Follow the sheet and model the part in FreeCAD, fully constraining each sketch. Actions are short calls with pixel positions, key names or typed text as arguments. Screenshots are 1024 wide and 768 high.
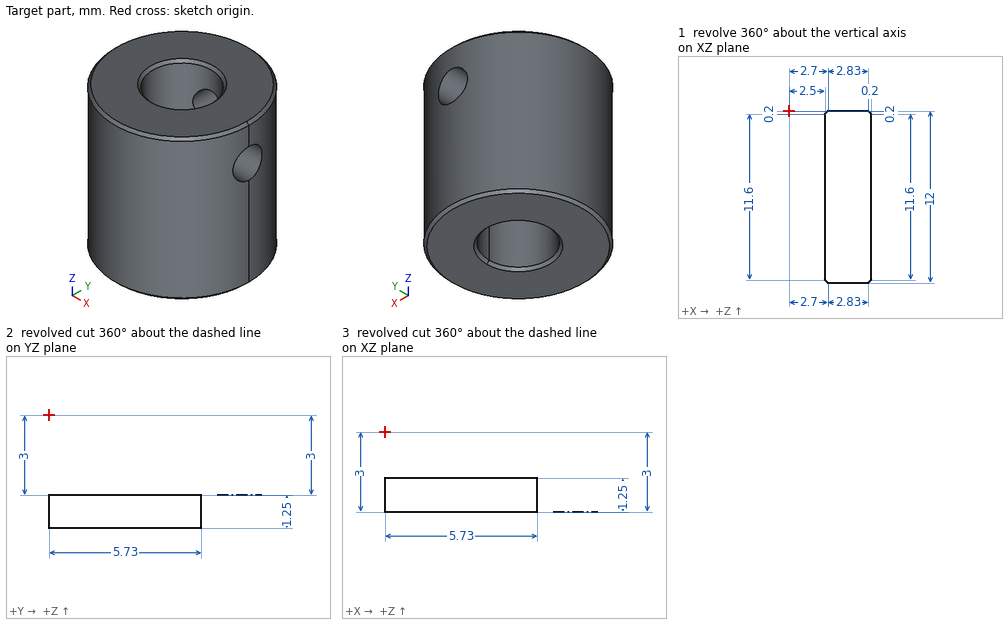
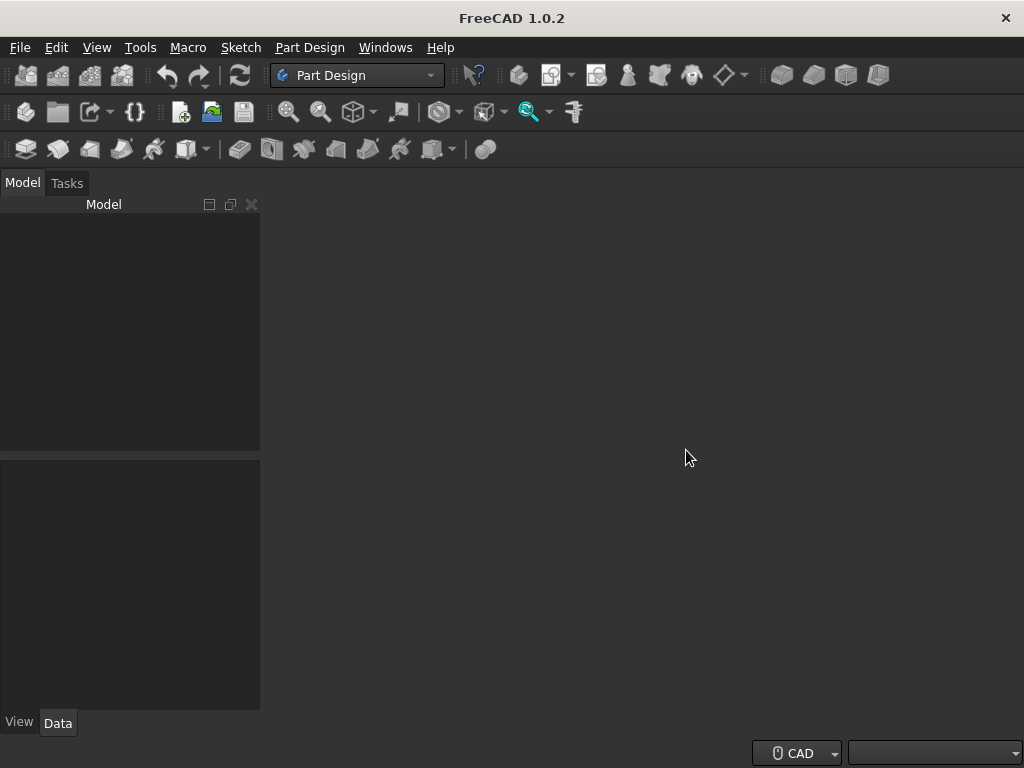
key(ctrl+n)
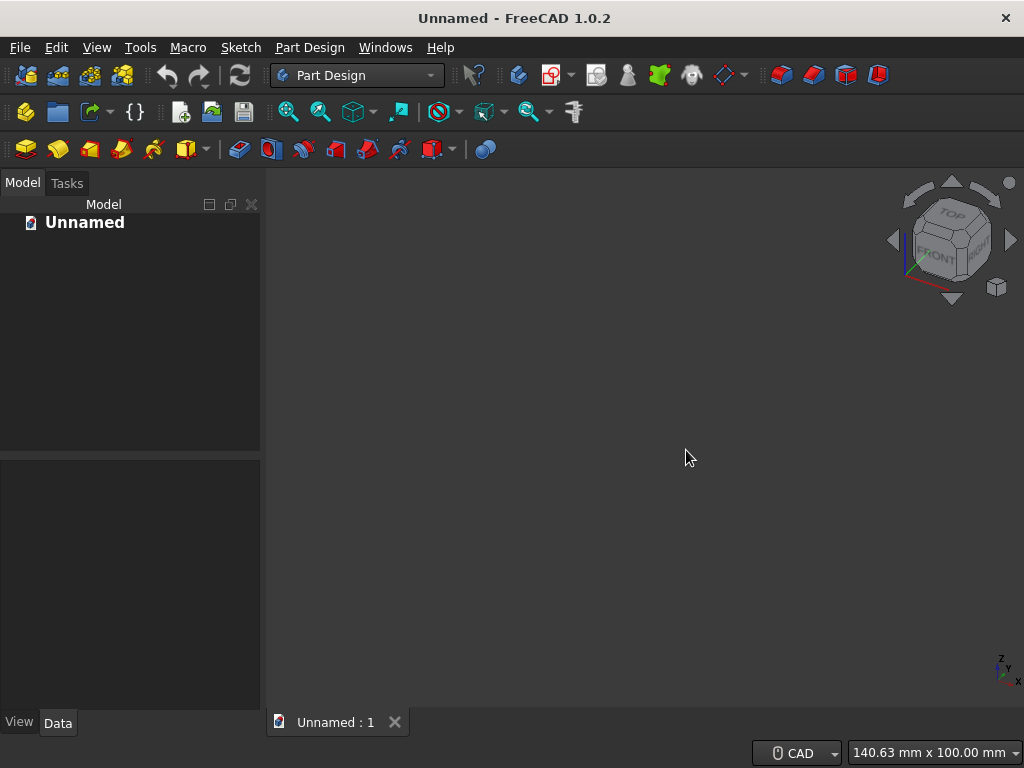
click(552, 76)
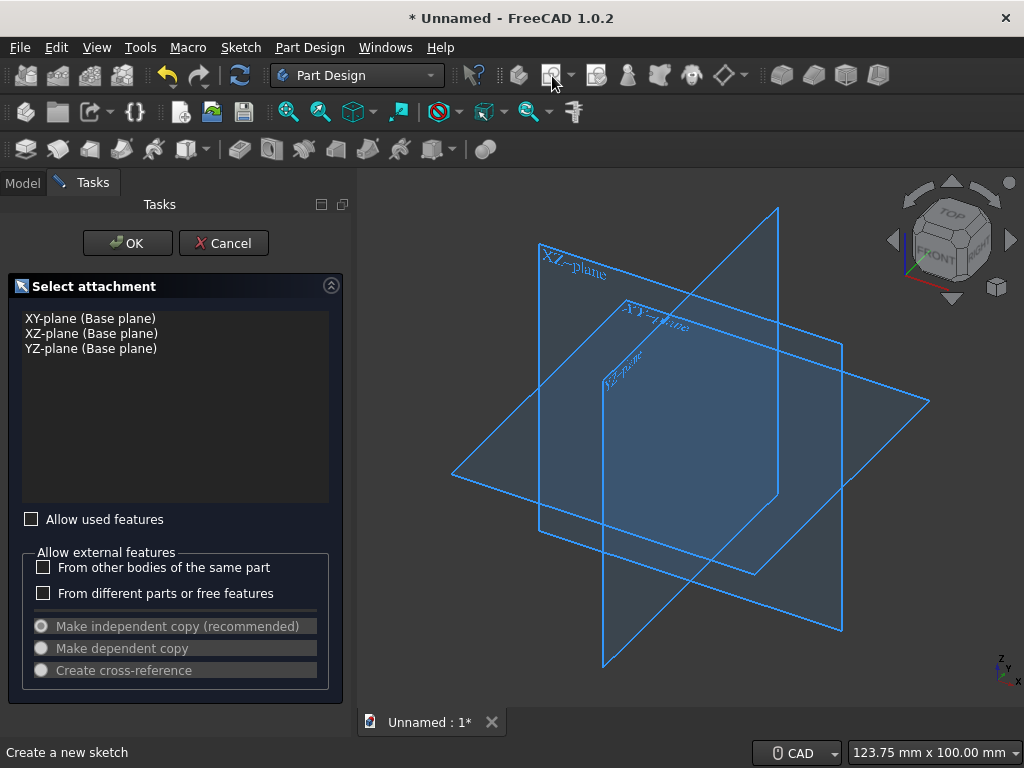
click(82, 334)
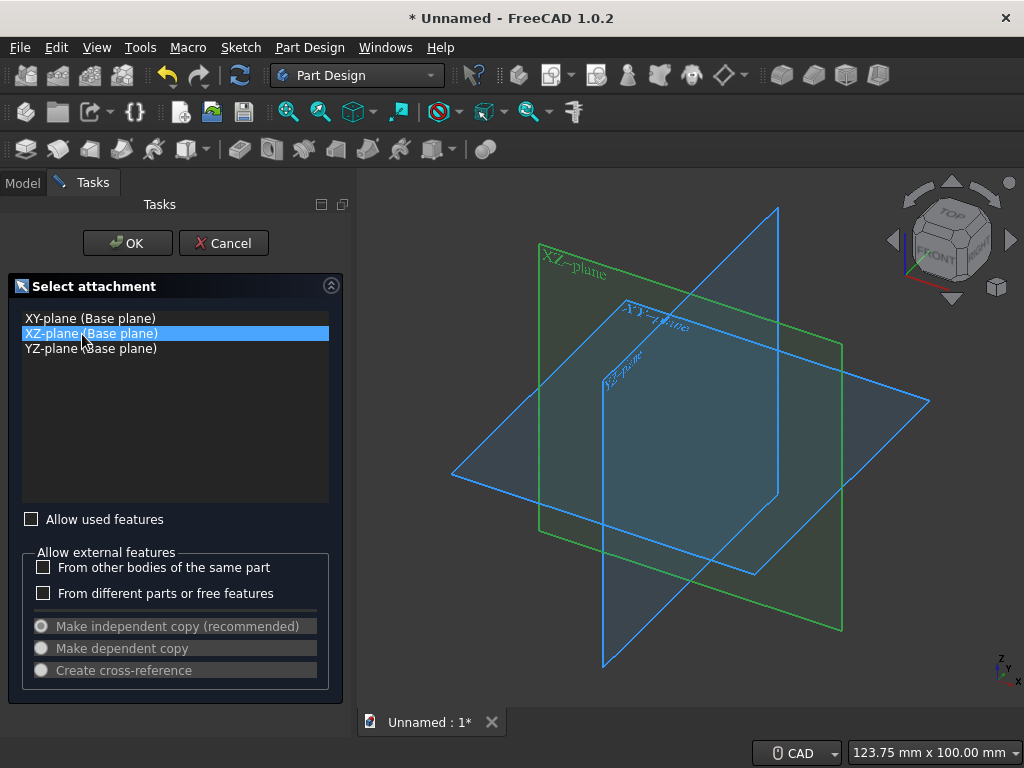
click(128, 243)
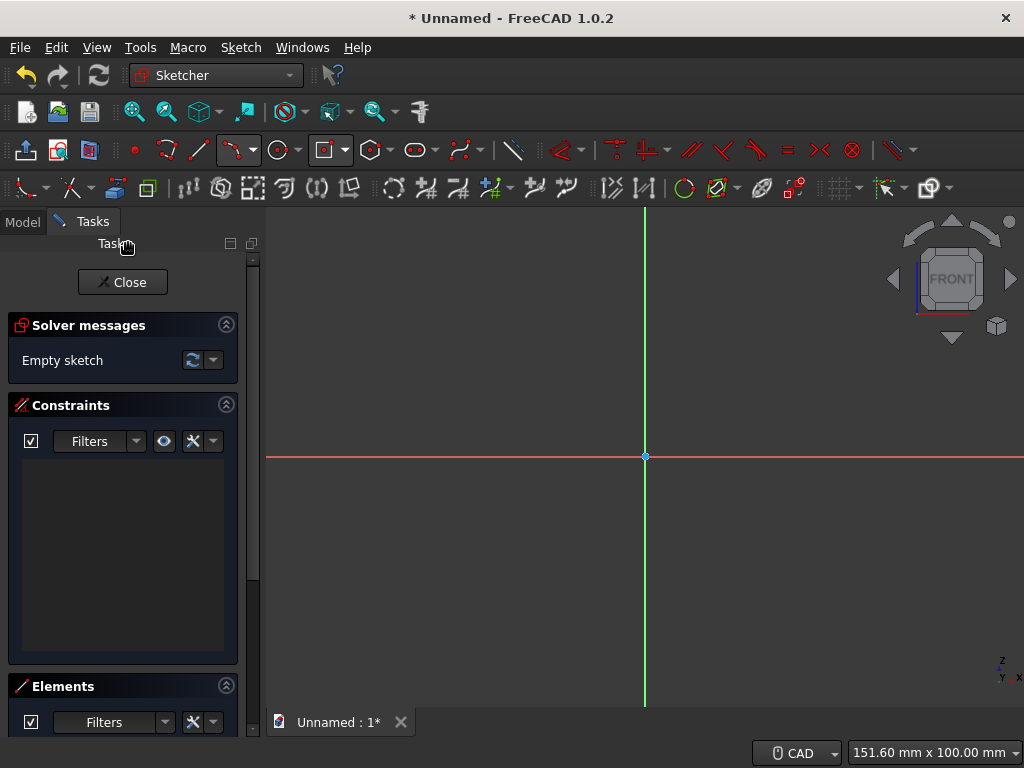
scroll(680, 495, up, 8)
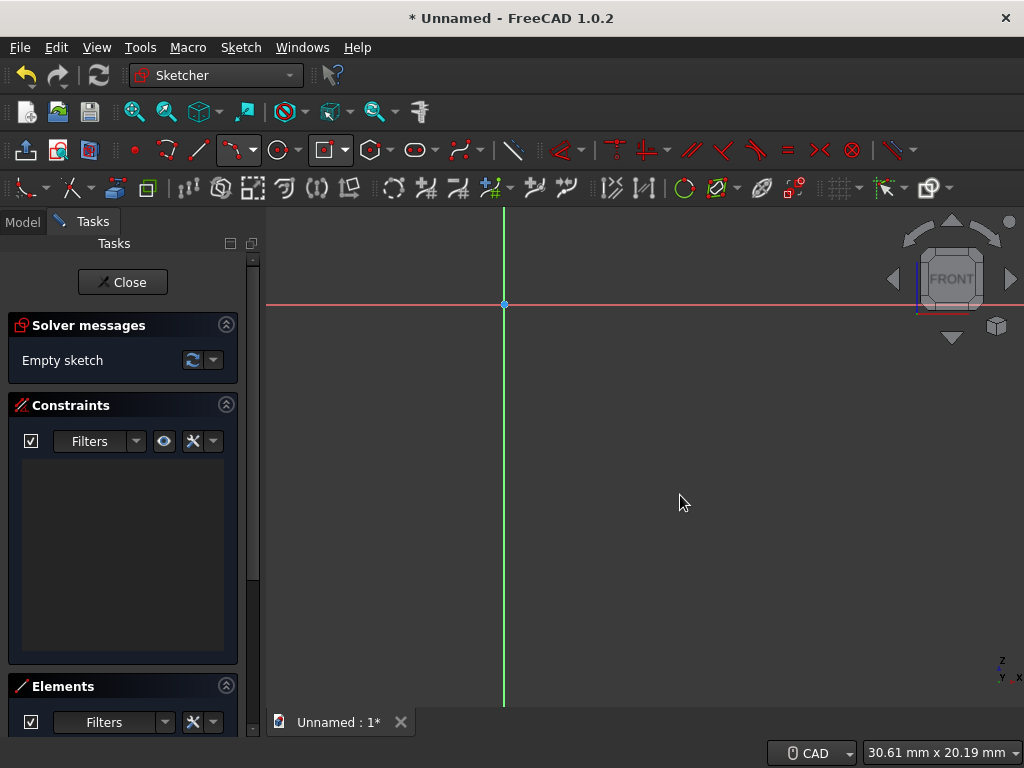
click(168, 150)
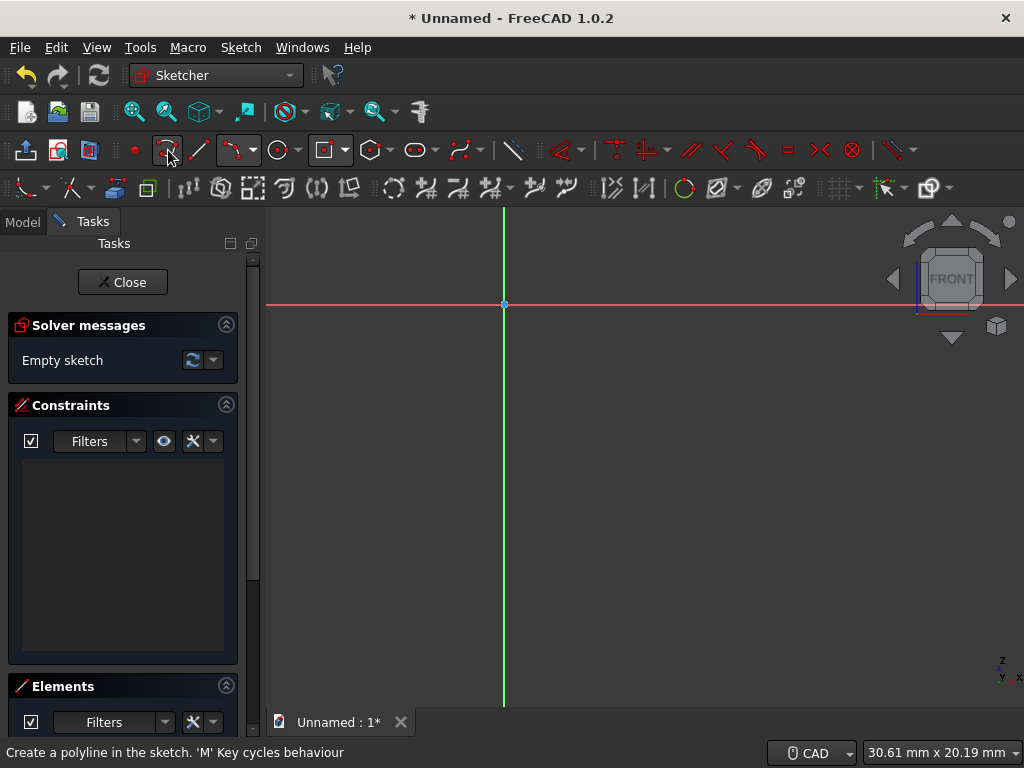
scroll(566, 309, up, 6)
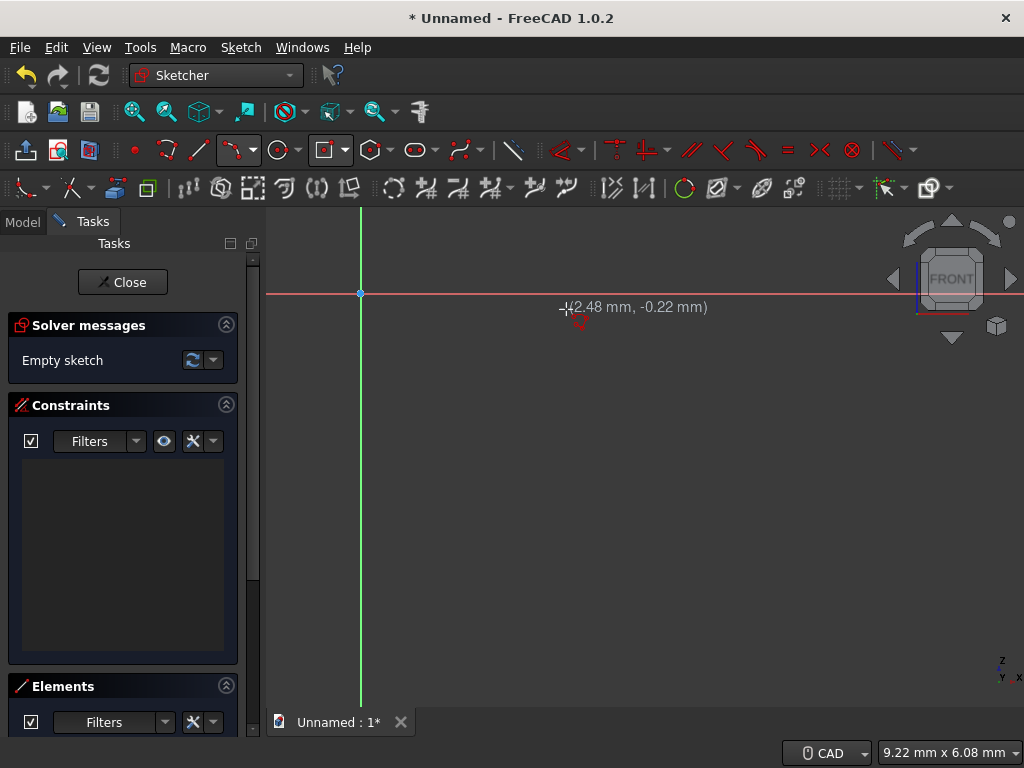
click(566, 310)
click(583, 294)
click(816, 303)
click(832, 310)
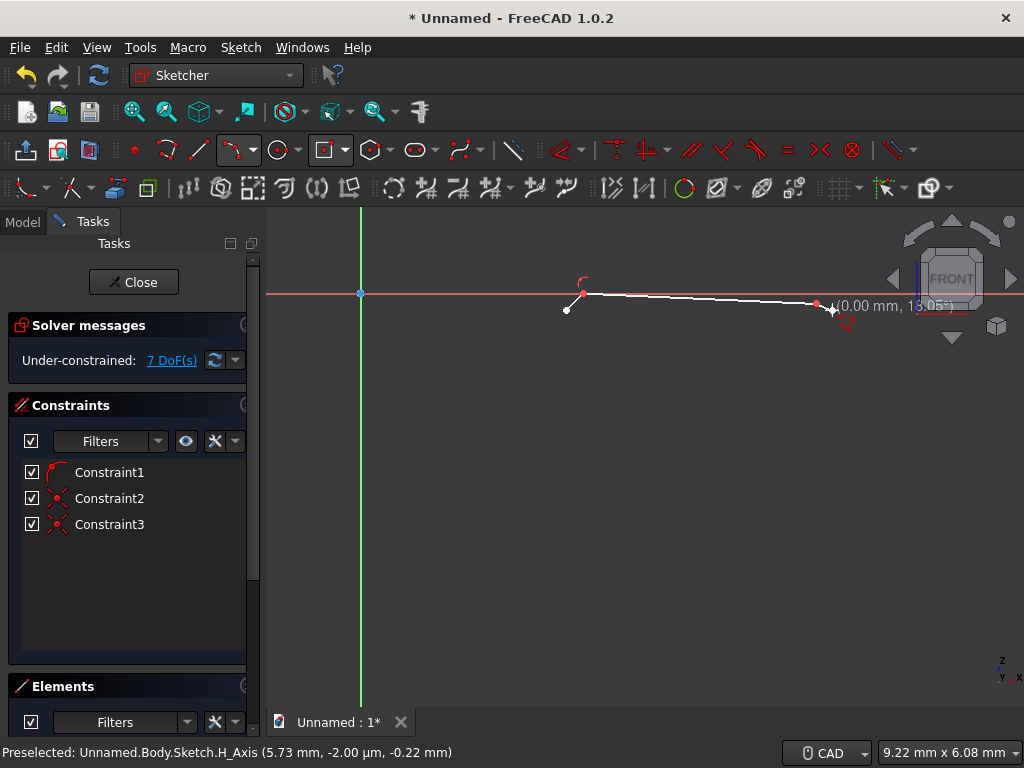
scroll(568, 315, down, 6)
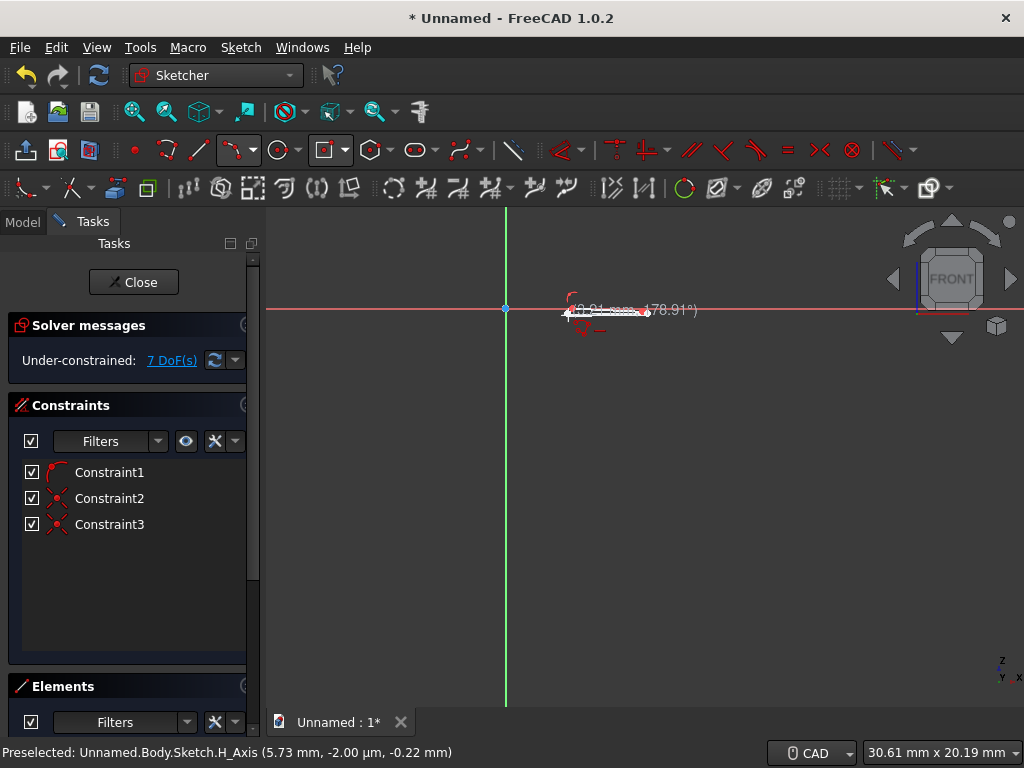
click(648, 601)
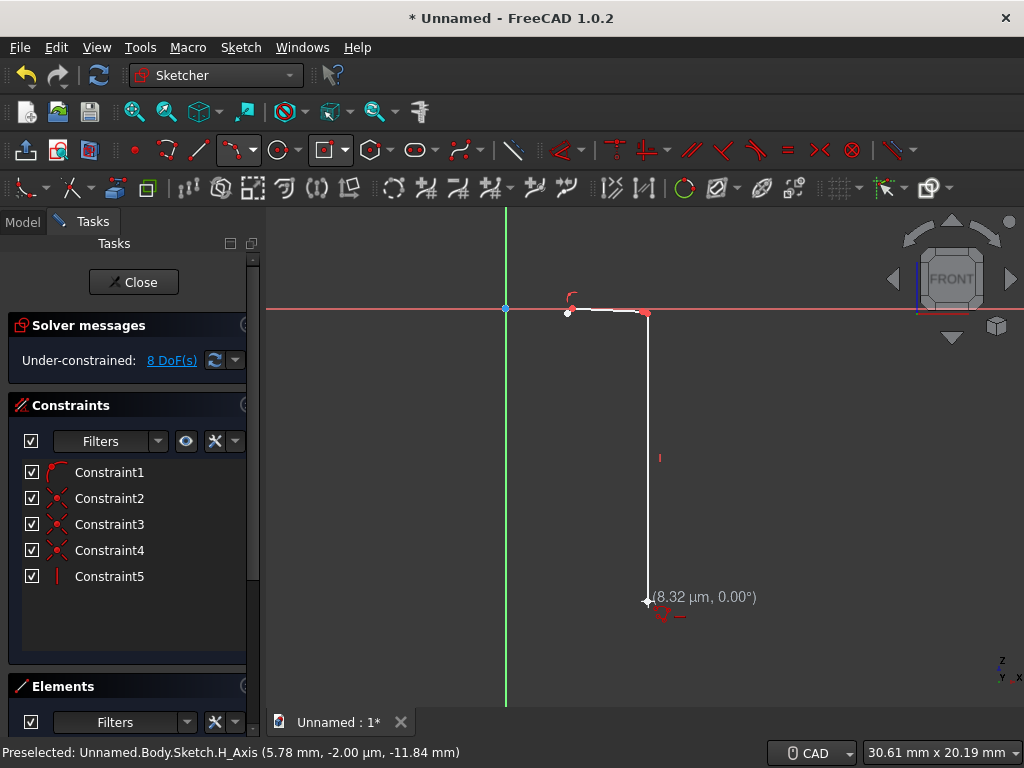
scroll(643, 606, up, 5)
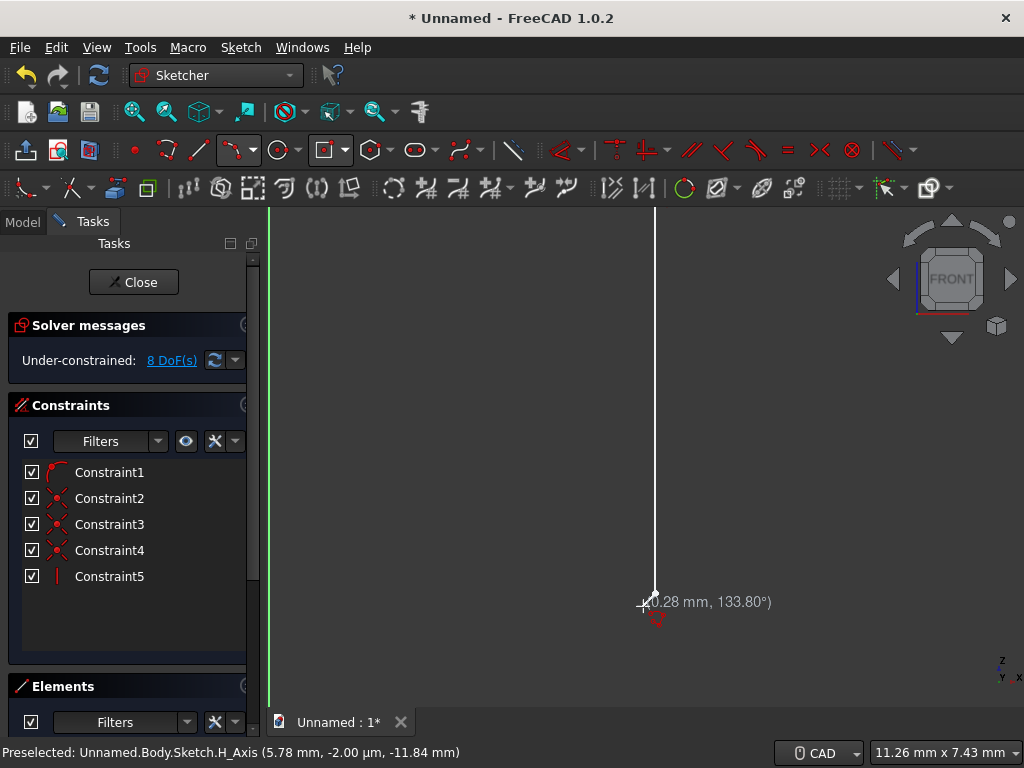
click(642, 604)
click(451, 604)
click(438, 591)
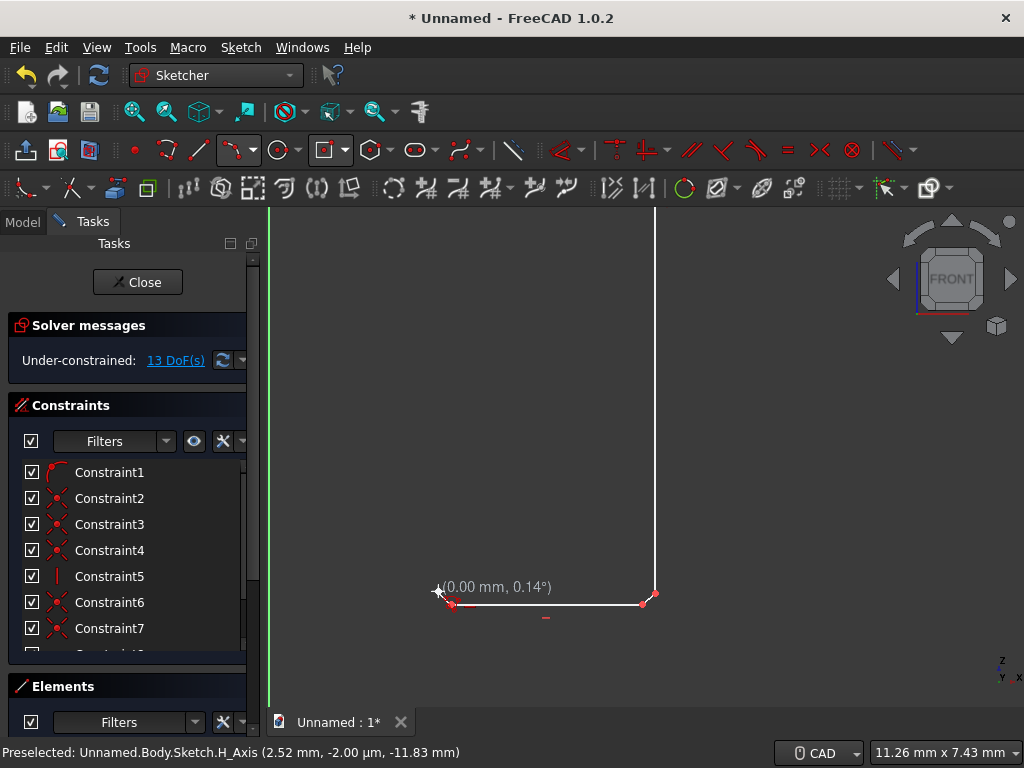
scroll(643, 606, down, 5)